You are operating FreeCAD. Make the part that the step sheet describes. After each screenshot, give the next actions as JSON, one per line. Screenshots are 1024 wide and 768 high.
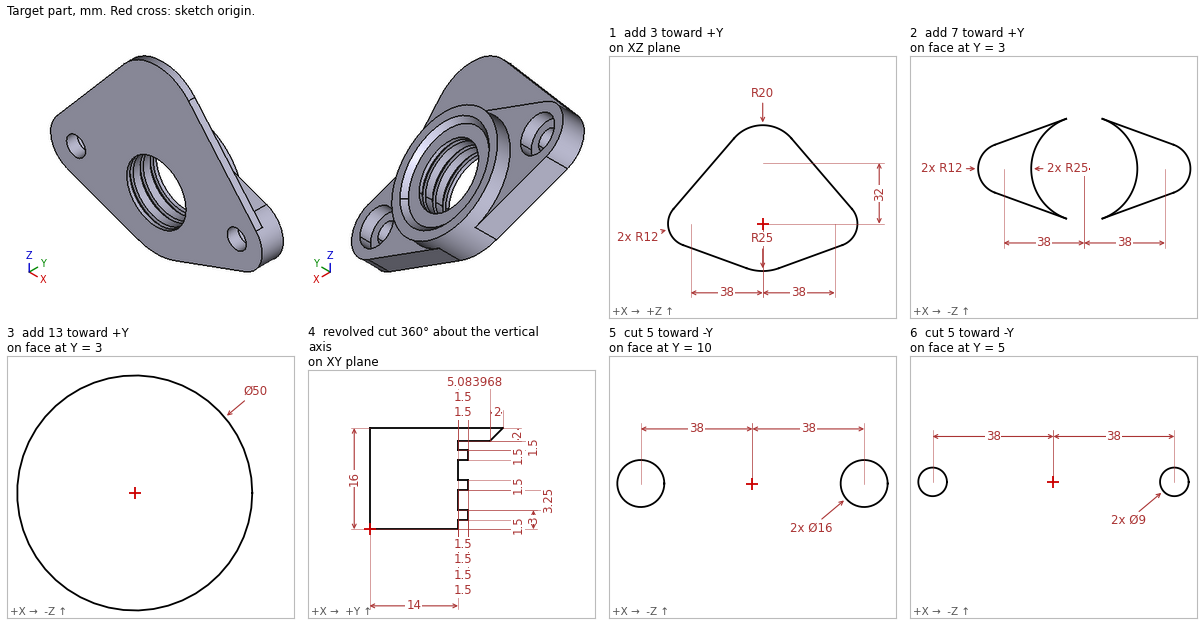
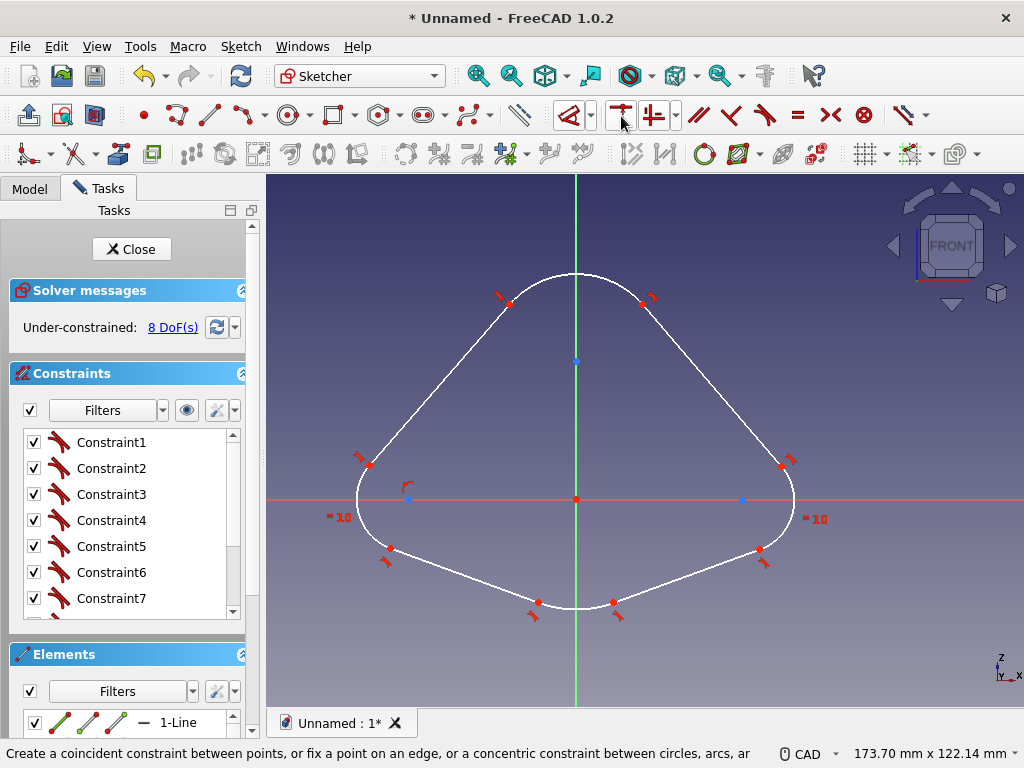
{"action": "left_click", "coordinate": [576, 362]}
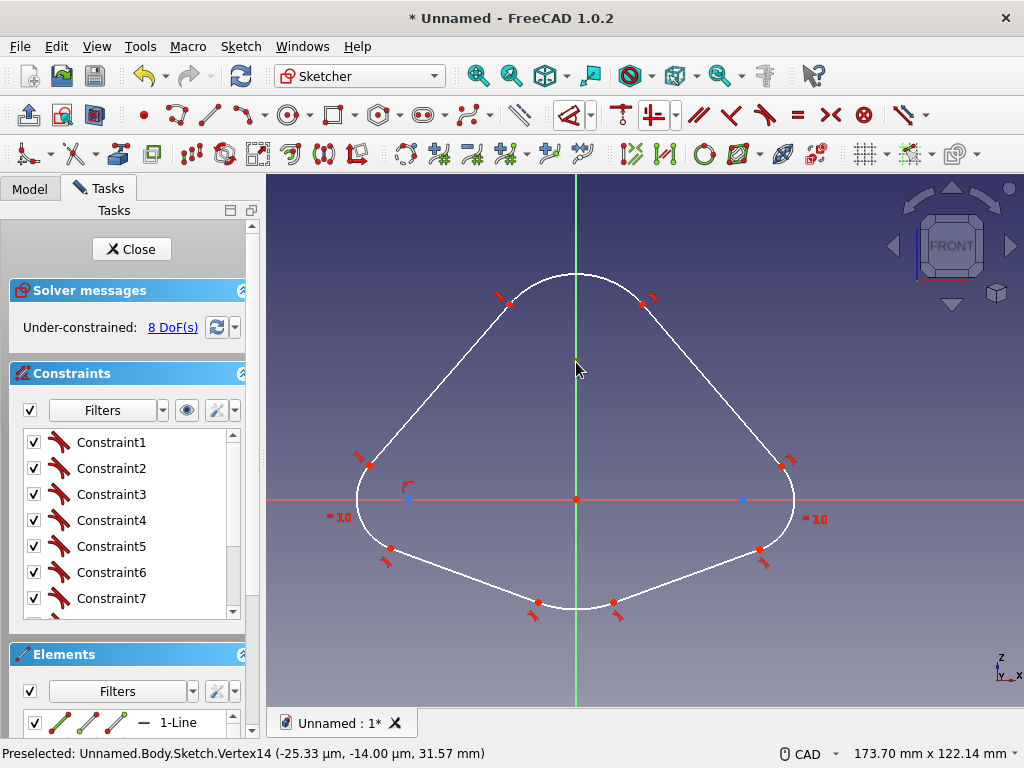
{"action": "left_click", "coordinate": [576, 645]}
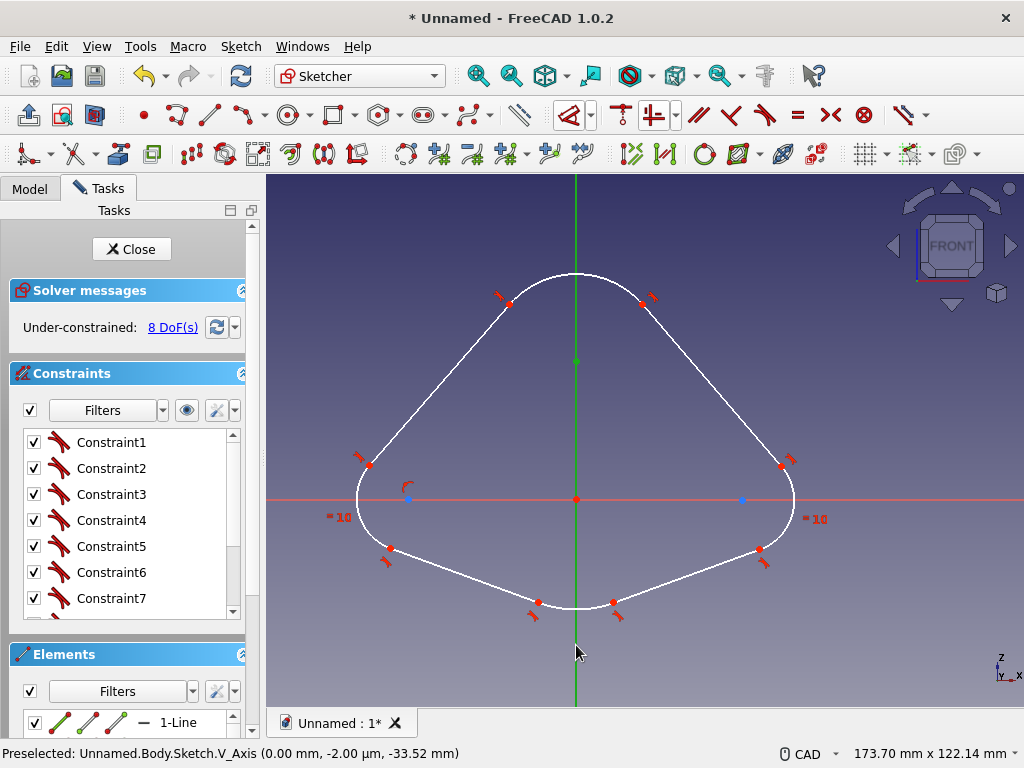
{"action": "left_click", "coordinate": [621, 116]}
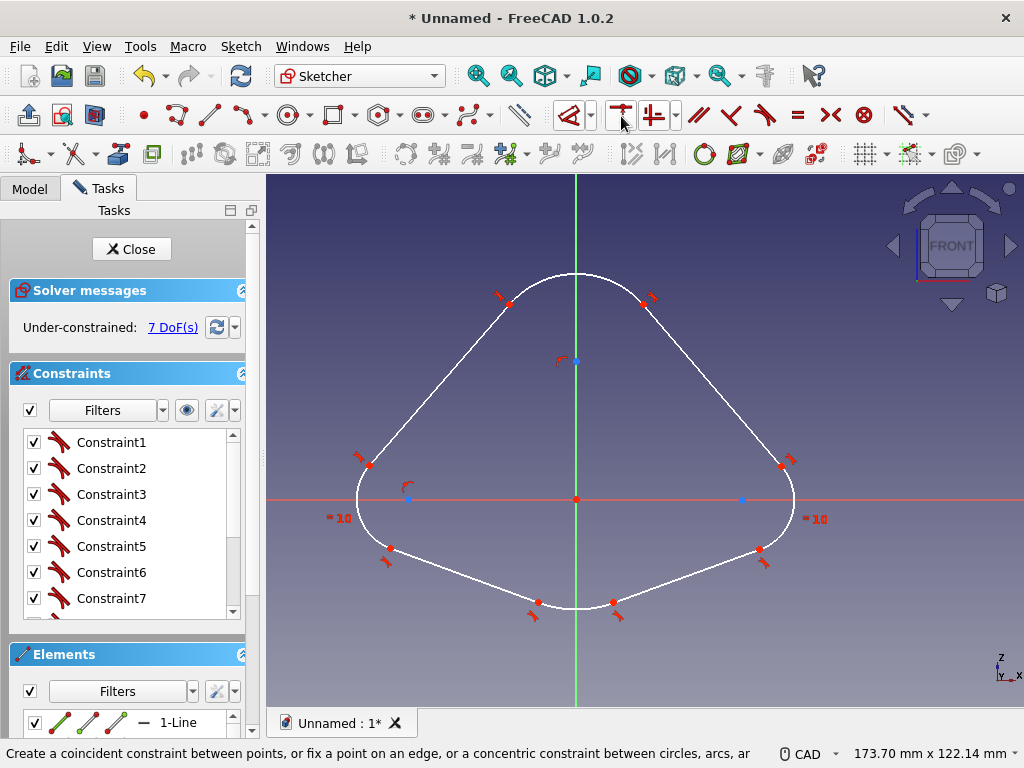
{"action": "left_click", "coordinate": [742, 501]}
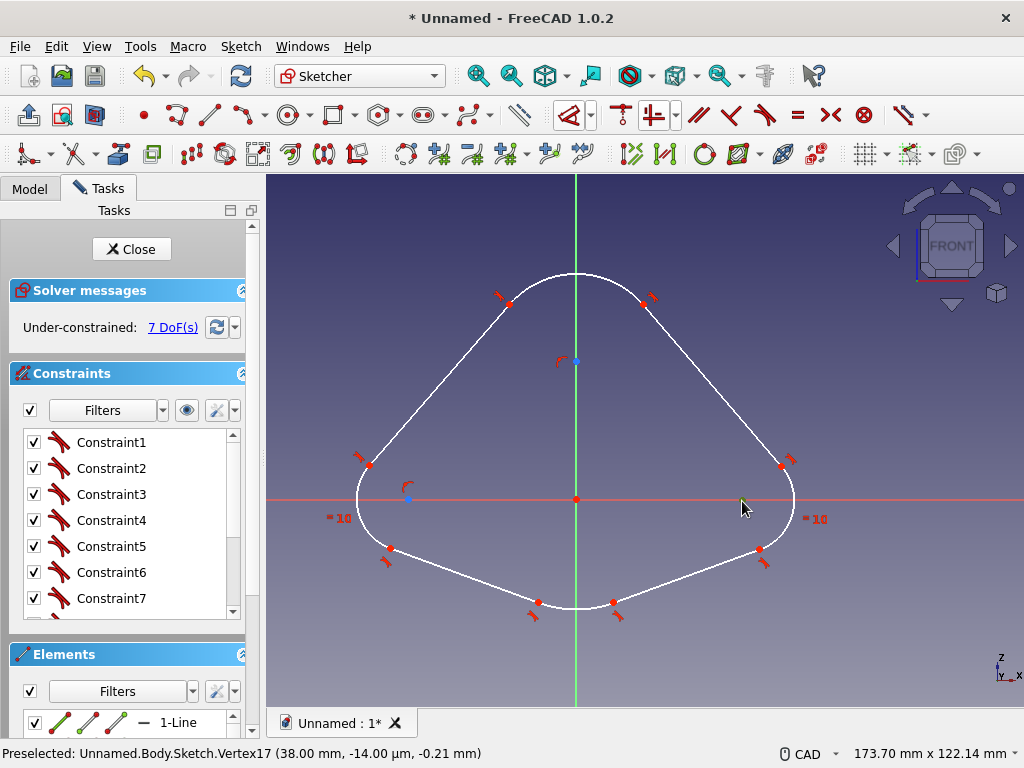
{"action": "left_click", "coordinate": [415, 500]}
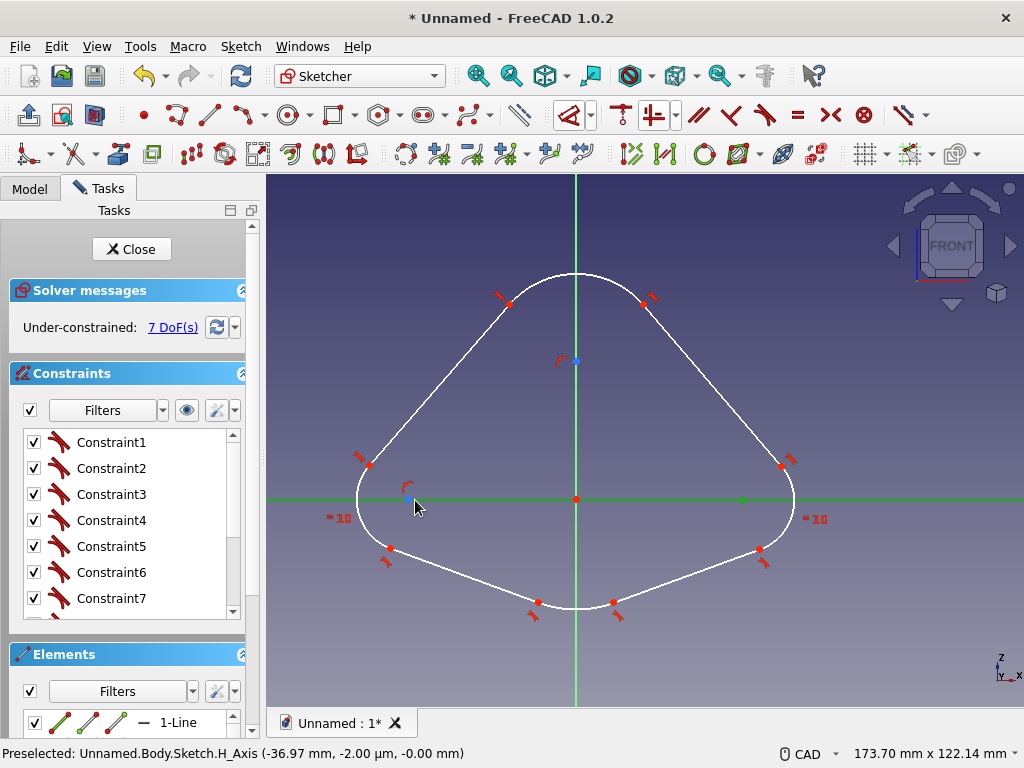
{"action": "left_click", "coordinate": [621, 116]}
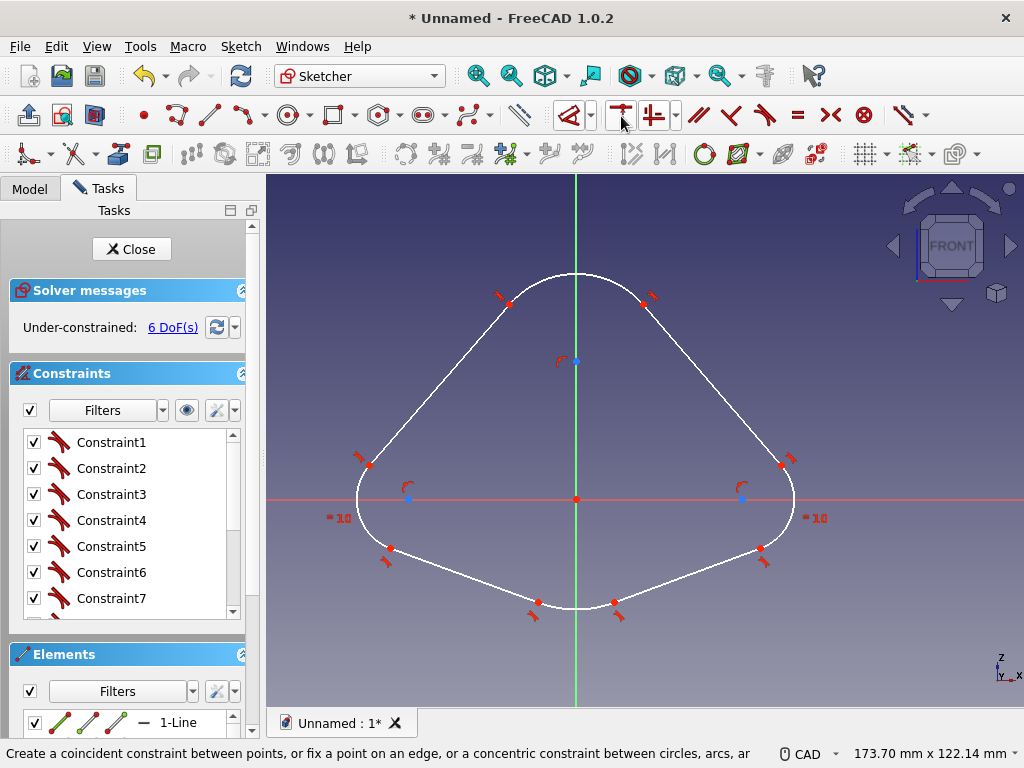
{"action": "left_click", "coordinate": [568, 116]}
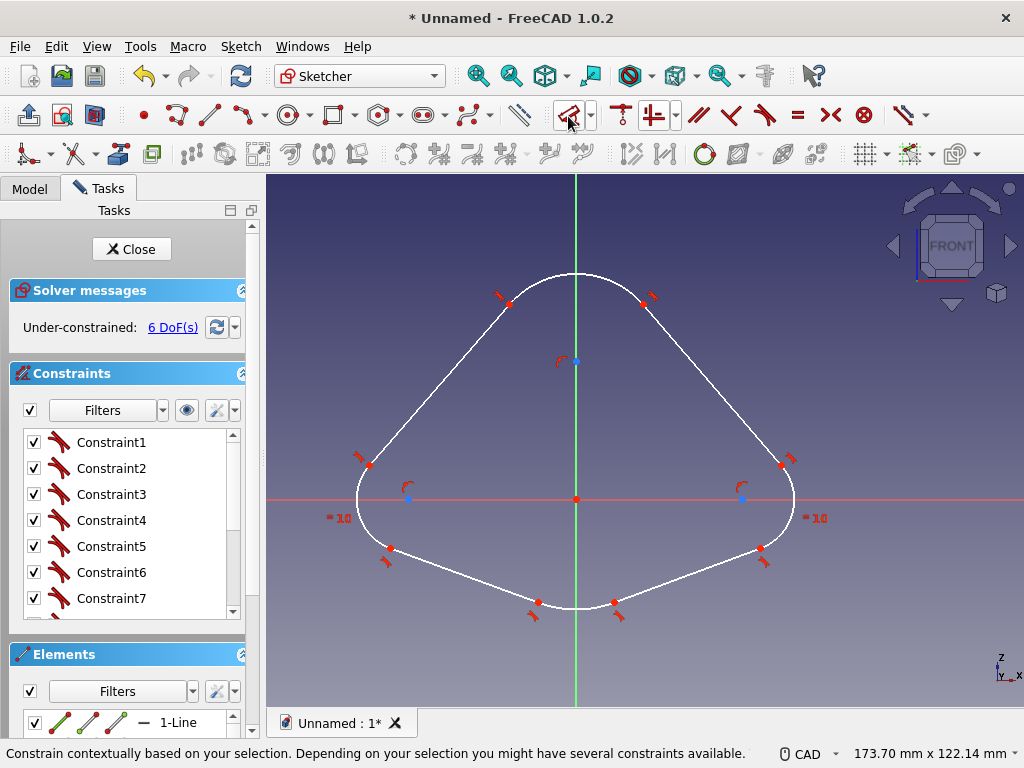
{"action": "left_click", "coordinate": [367, 531]}
{"action": "left_click", "coordinate": [341, 550]}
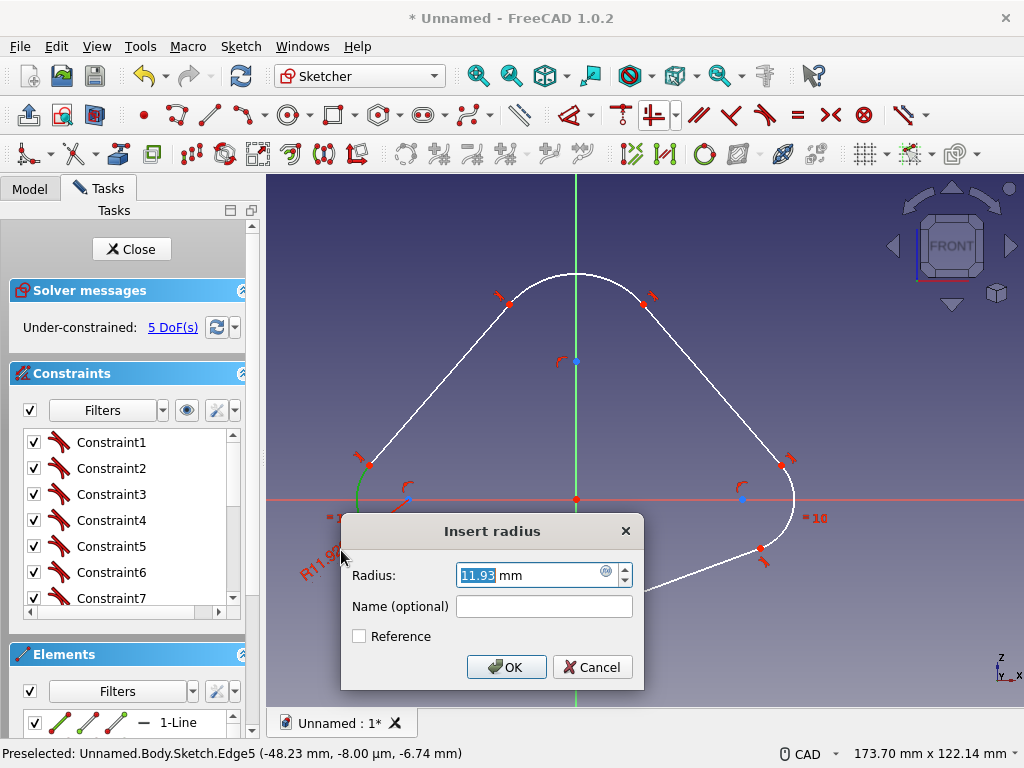
{"action": "type", "text": "12"}
{"action": "key", "text": "Return"}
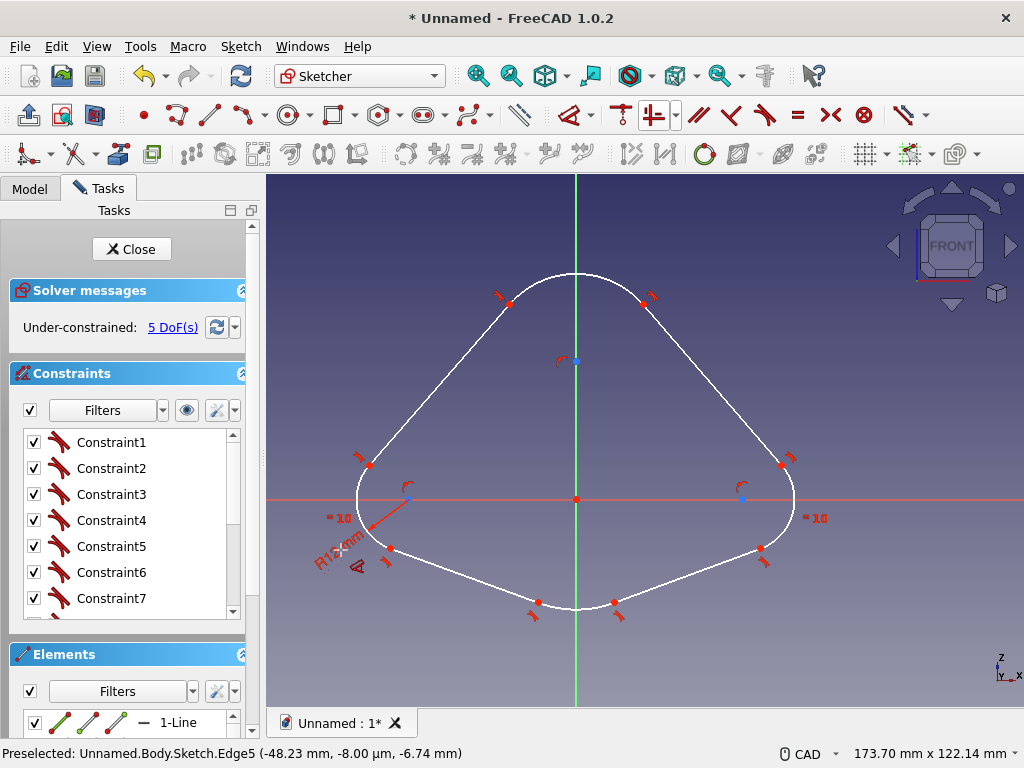
{"action": "left_click", "coordinate": [606, 279]}
{"action": "left_click", "coordinate": [617, 249]}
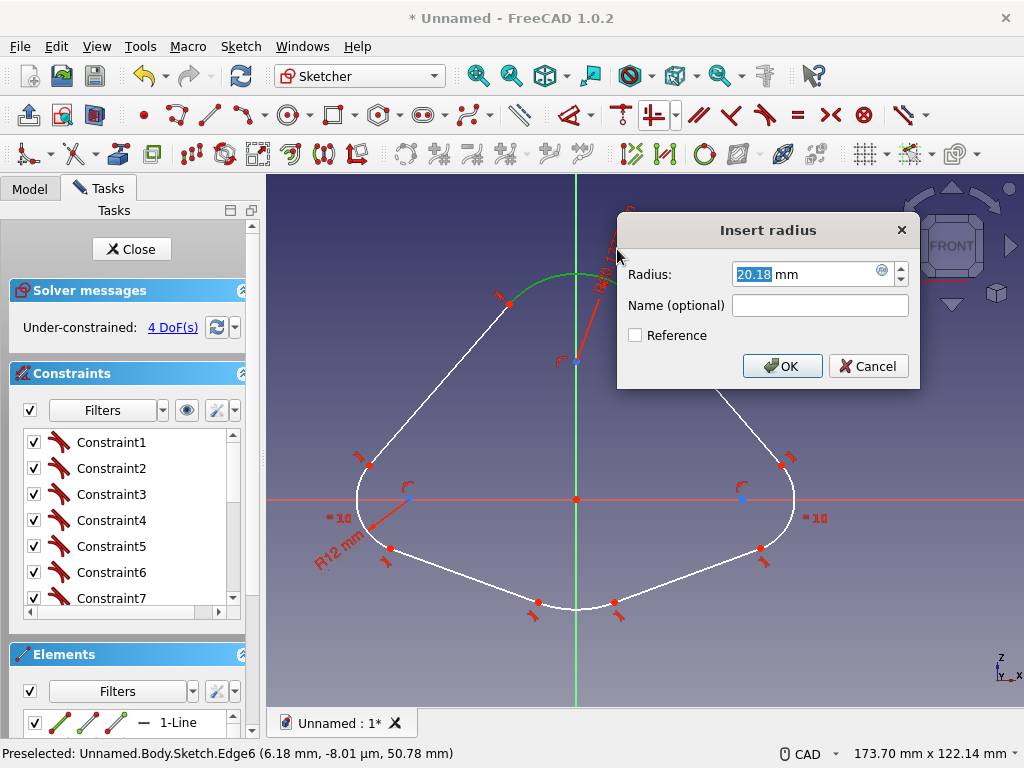
{"action": "type", "text": "20"}
{"action": "key", "text": "Return"}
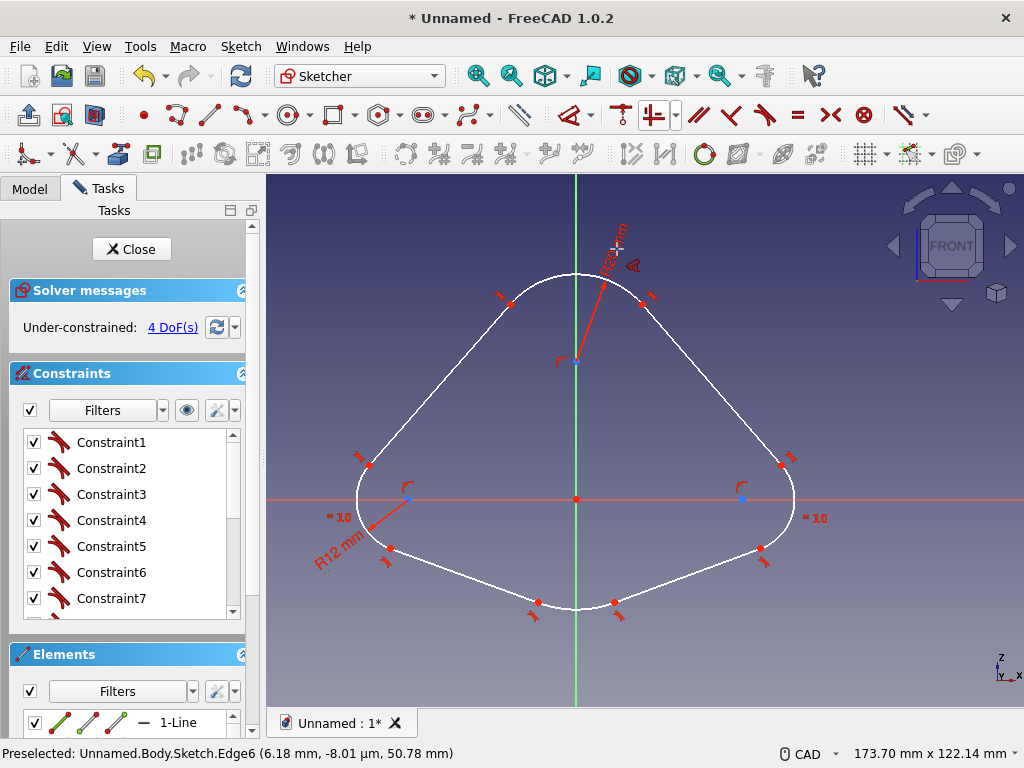
{"action": "left_click", "coordinate": [561, 609]}
{"action": "left_click", "coordinate": [557, 641]}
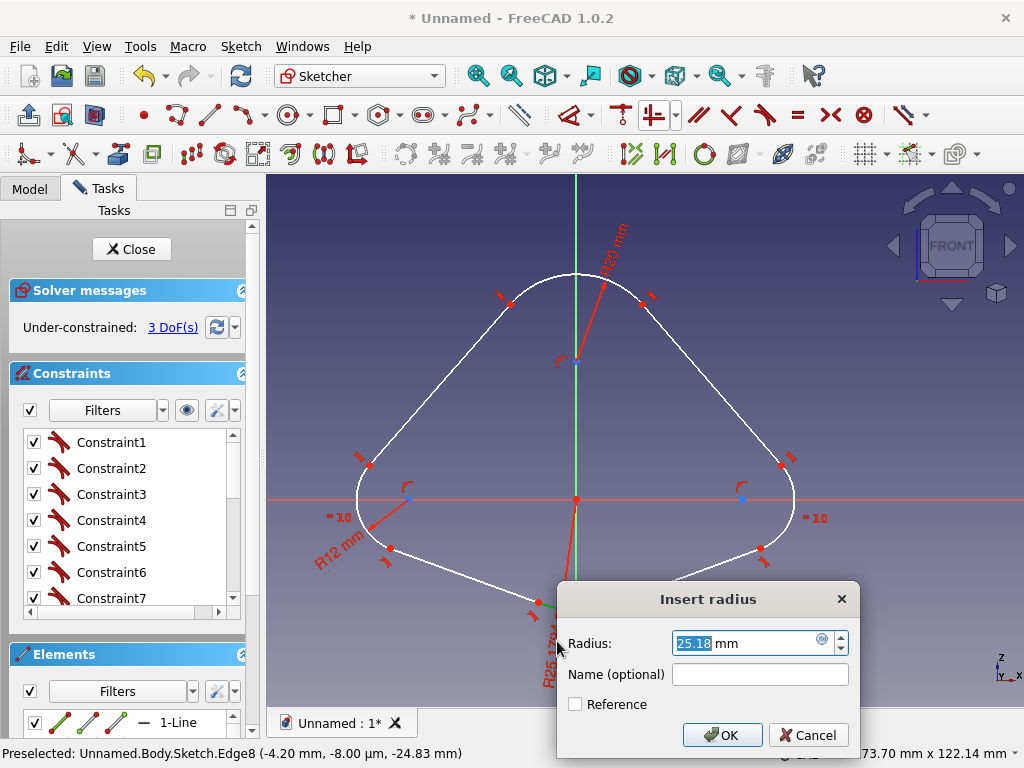
{"action": "type", "text": "25"}
{"action": "key", "text": "Return"}